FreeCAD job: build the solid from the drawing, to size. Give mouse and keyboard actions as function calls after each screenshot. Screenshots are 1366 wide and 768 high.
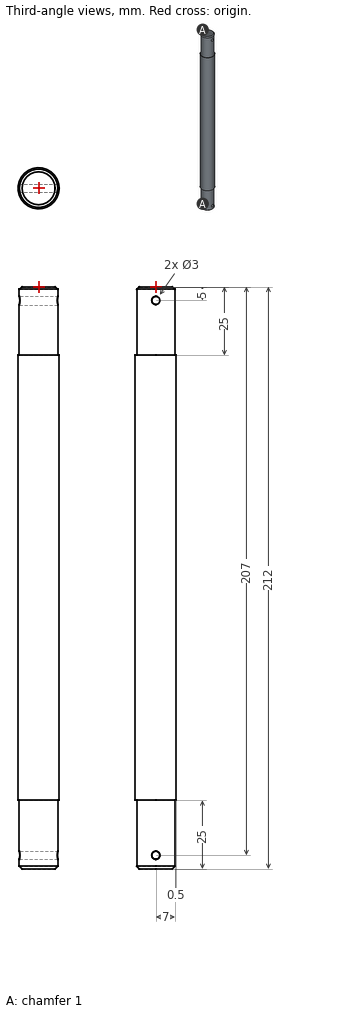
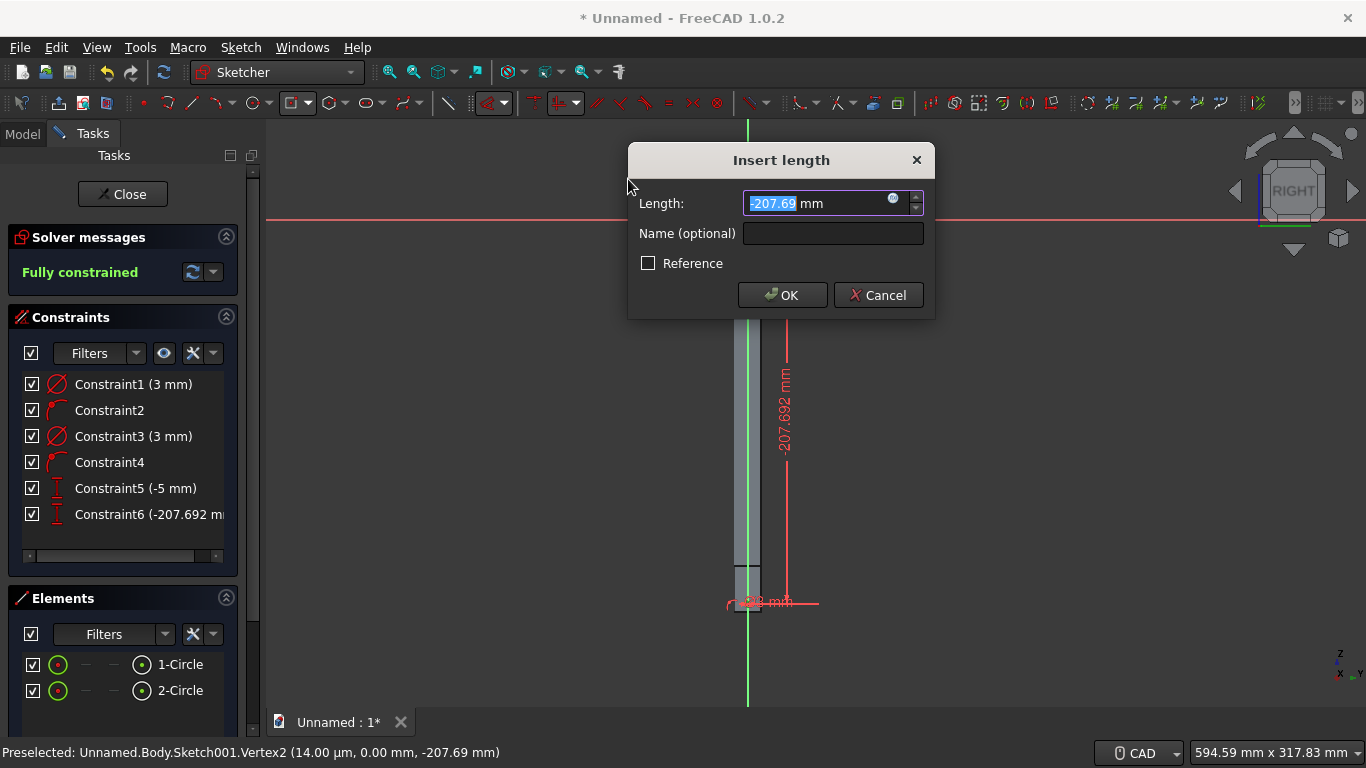
text(-207)
key(Return)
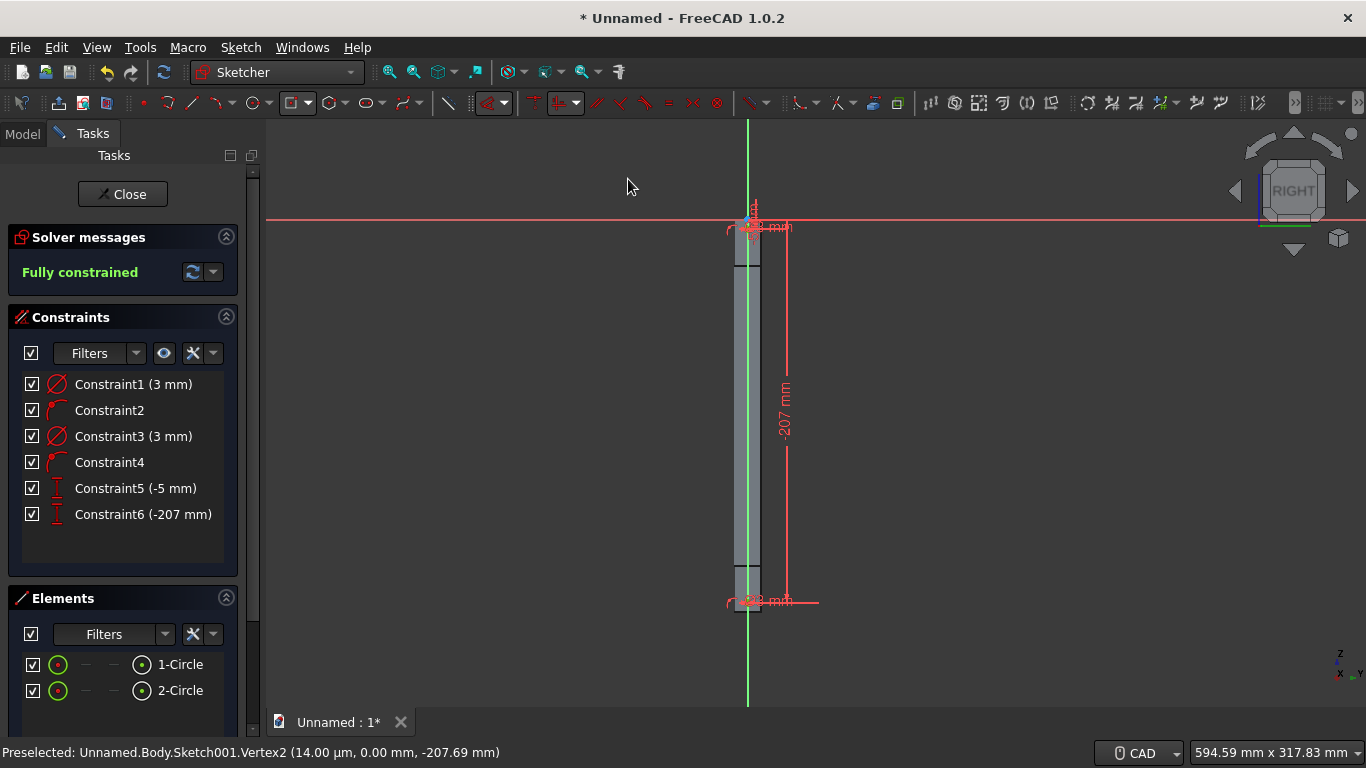
click(123, 194)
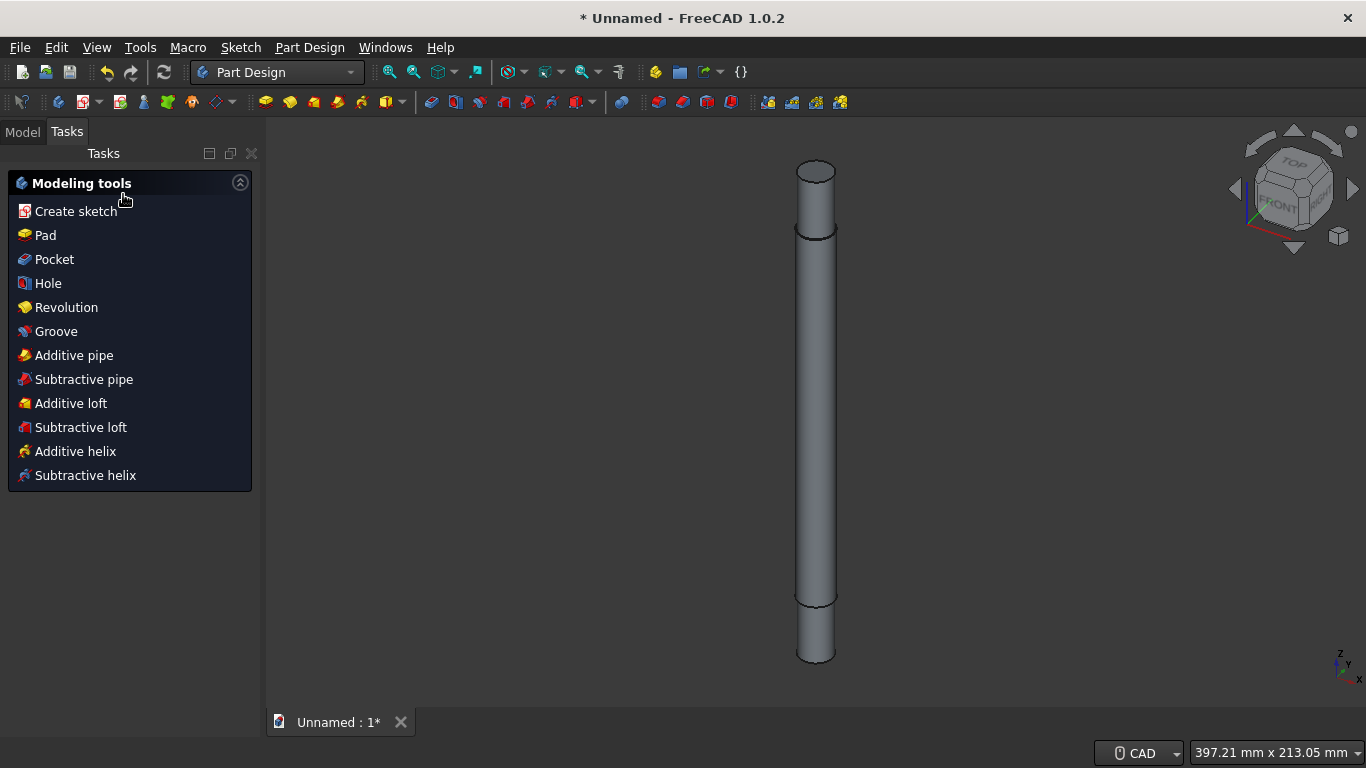
click(432, 102)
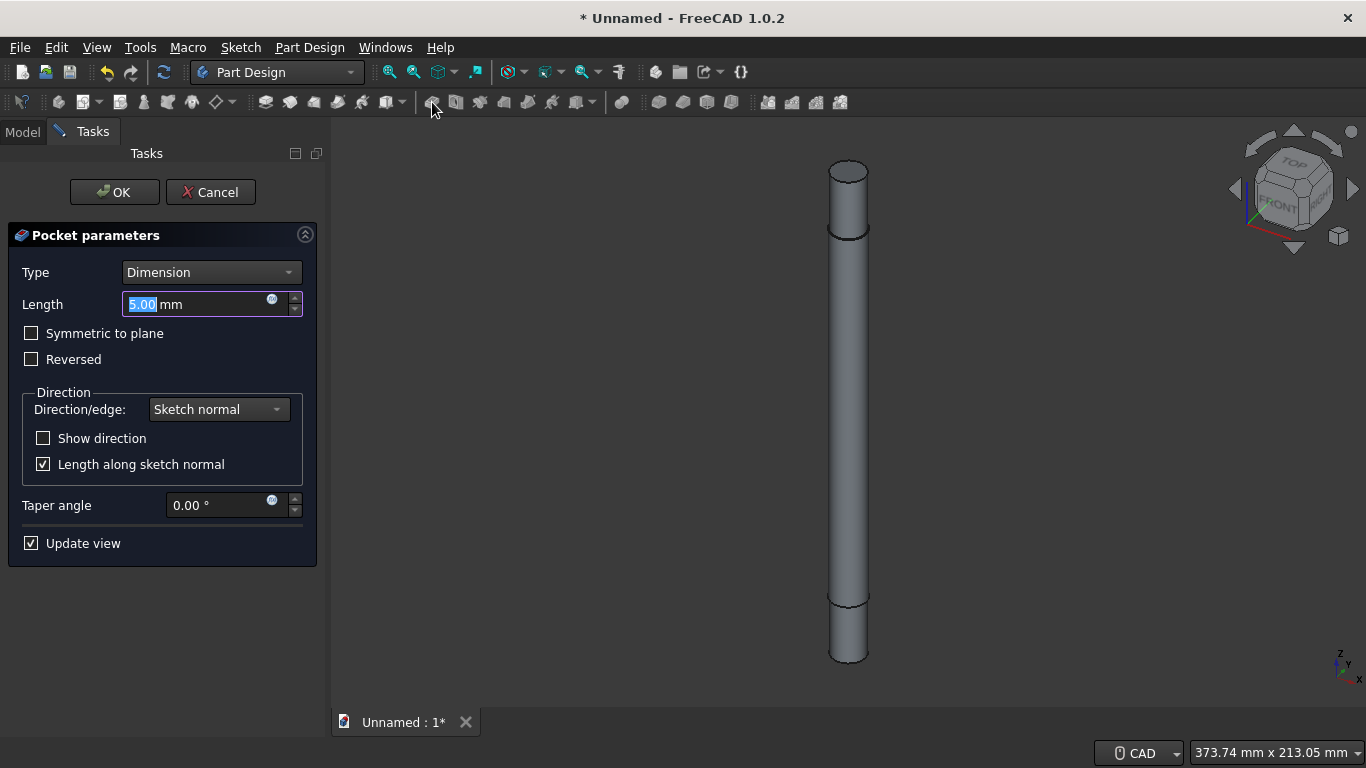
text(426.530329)
key(Tab)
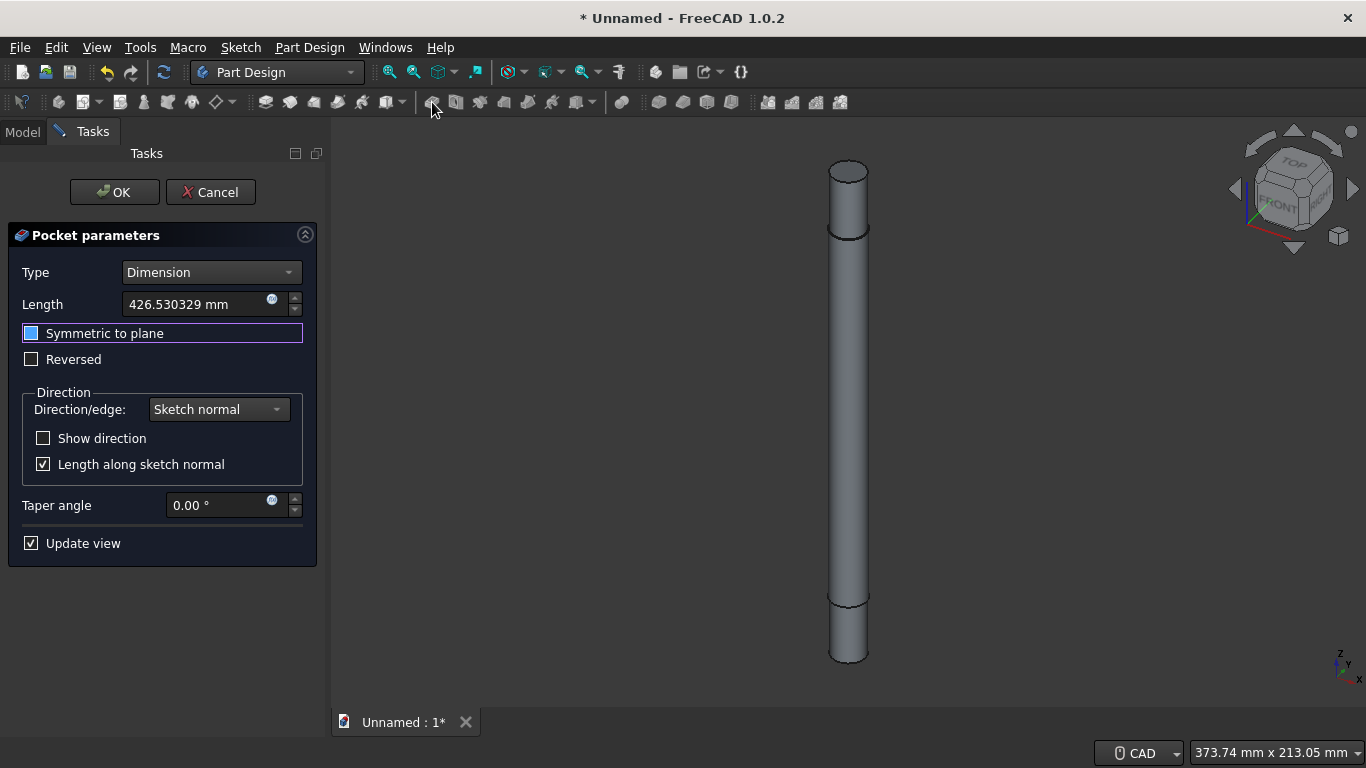
click(30, 333)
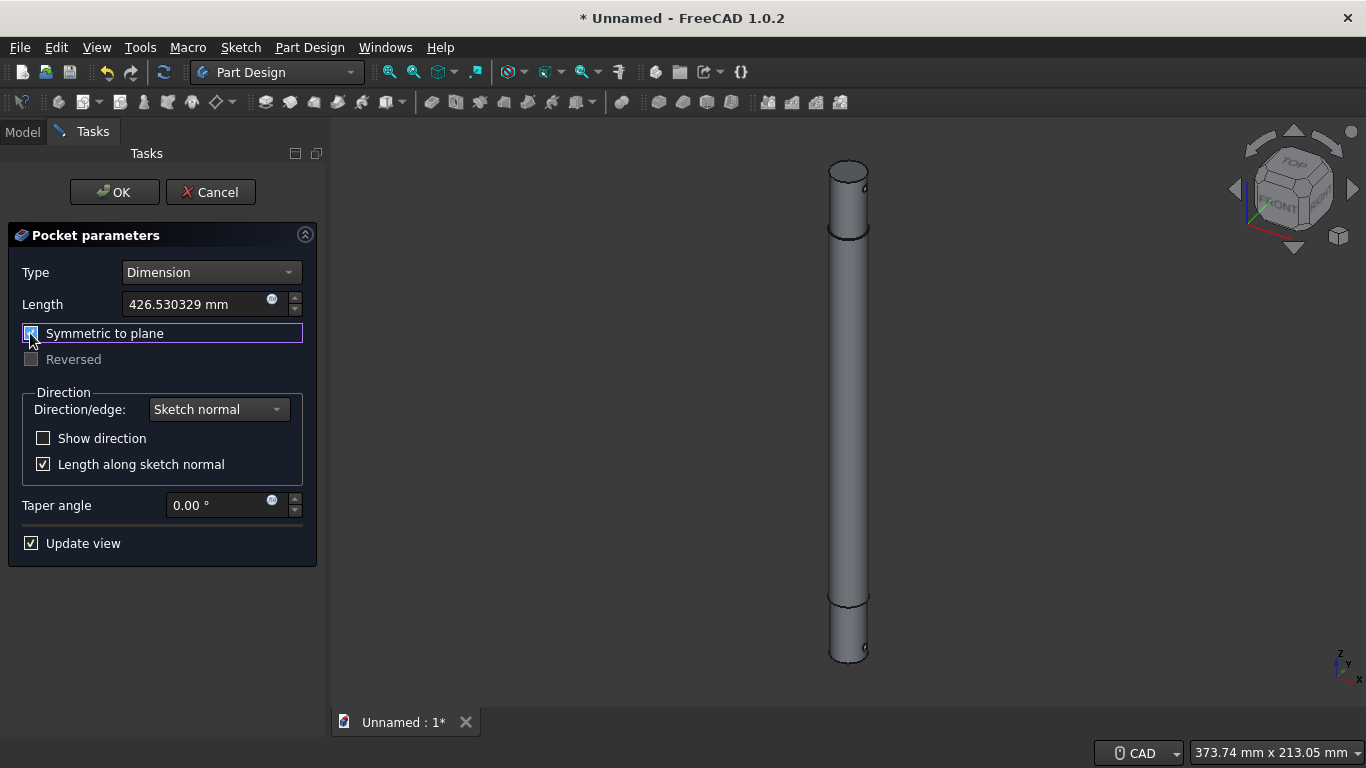
click(115, 192)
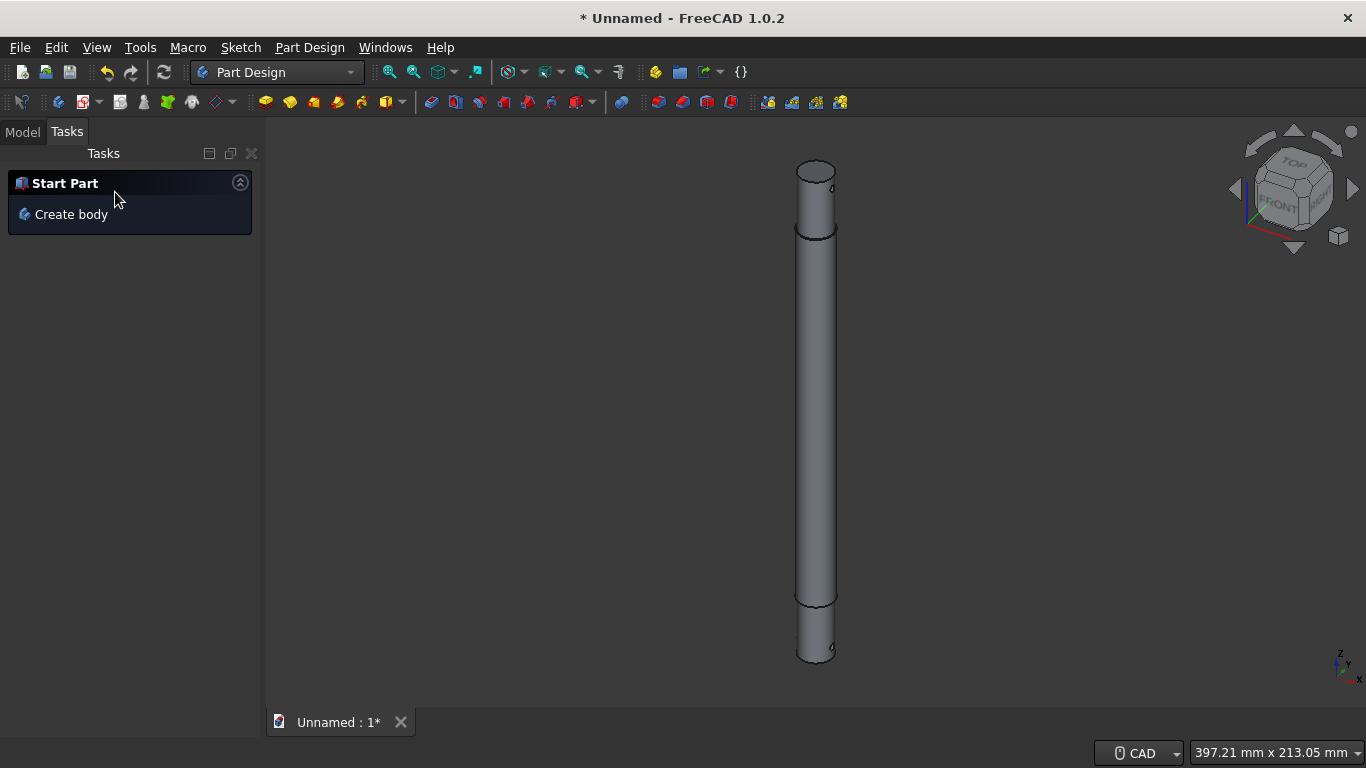
click(806, 180)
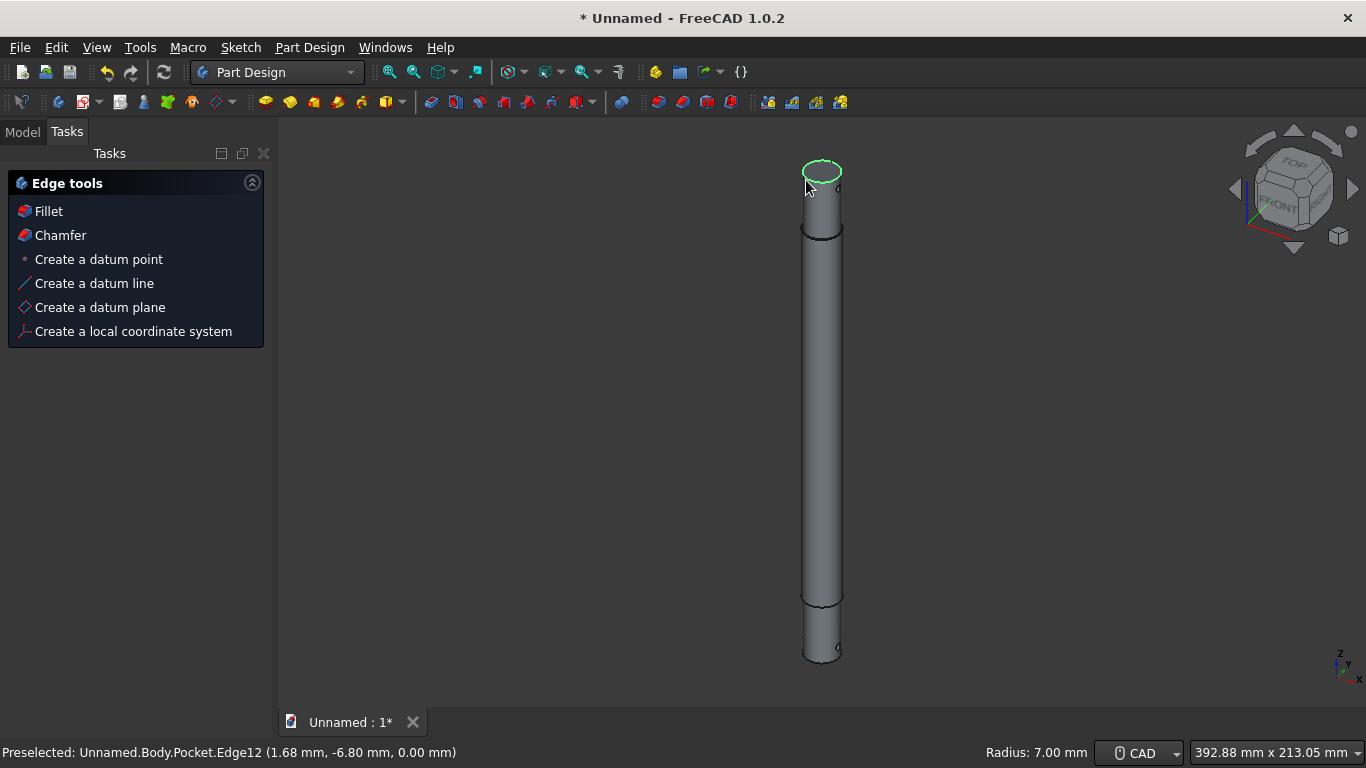
click(812, 661, ctrl)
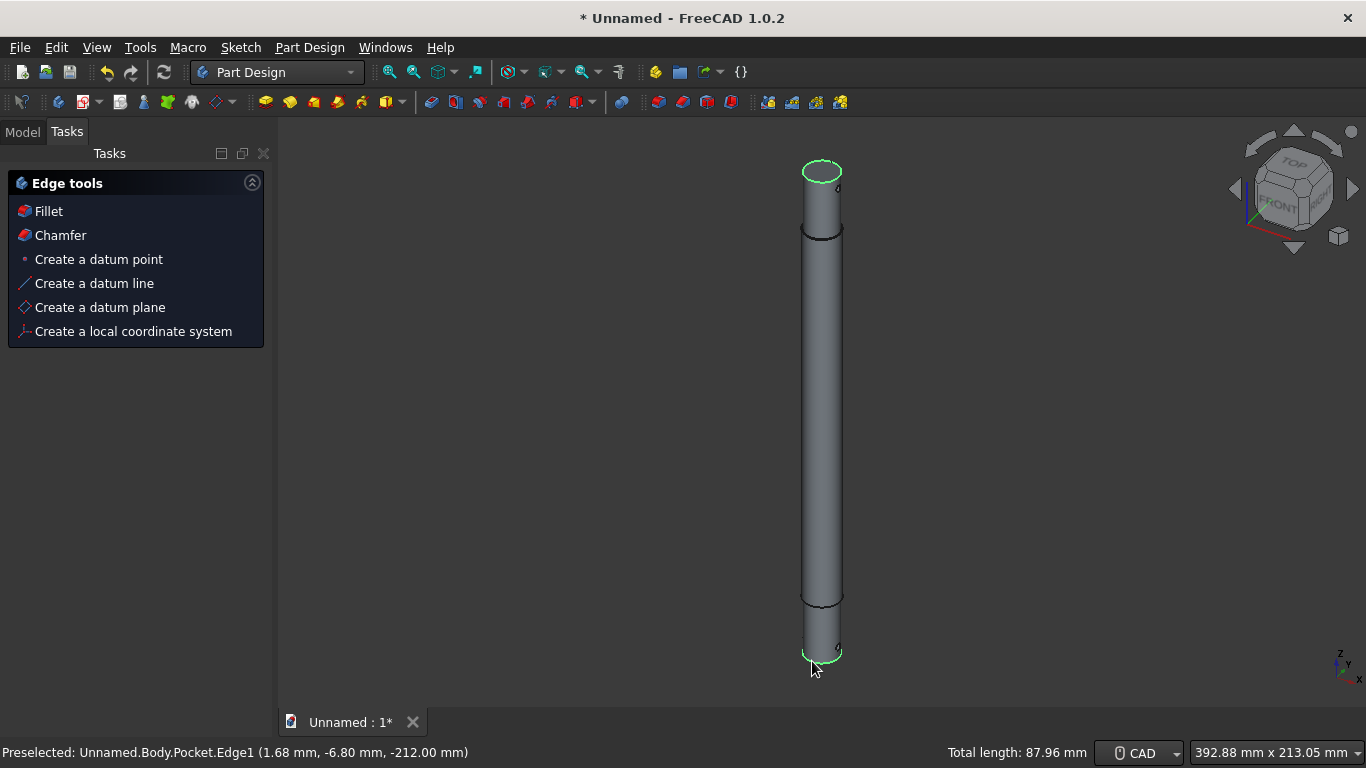
click(684, 102)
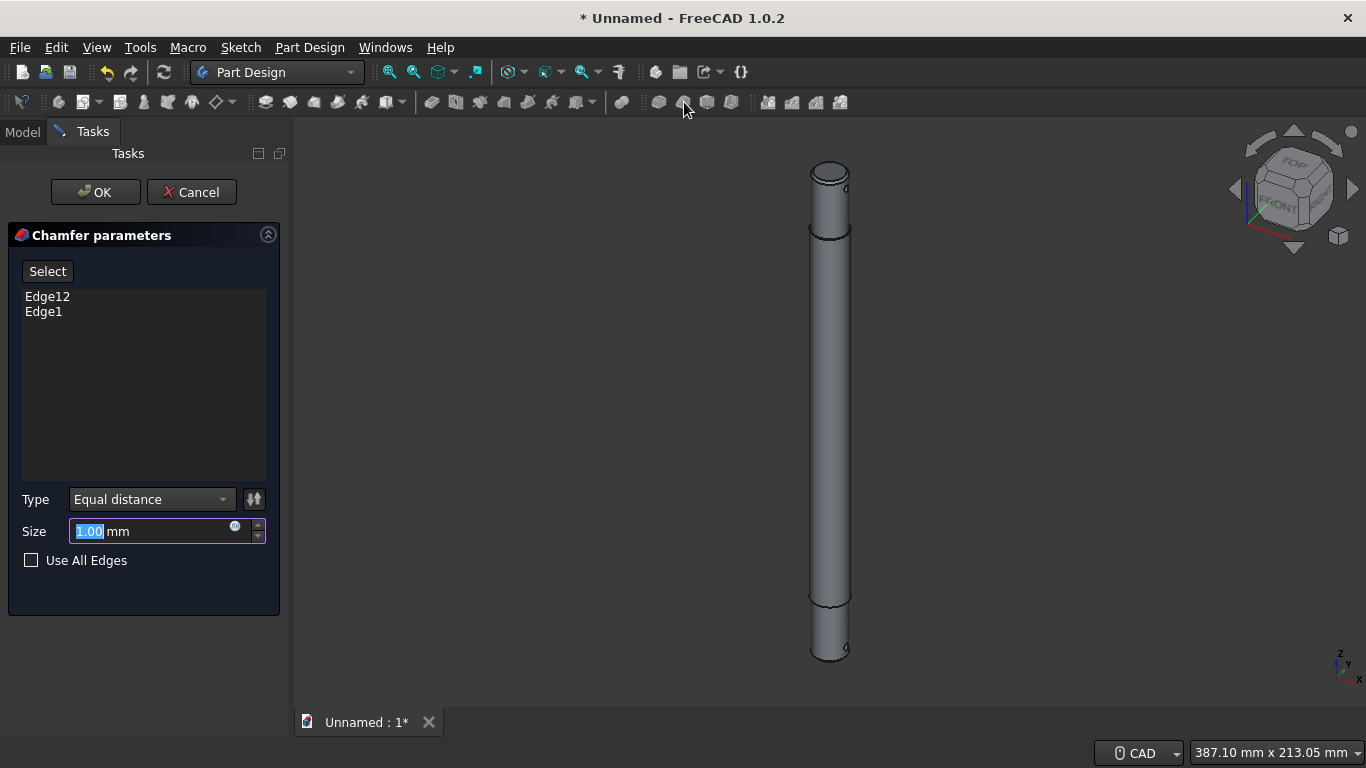
text(1)
key(Tab)